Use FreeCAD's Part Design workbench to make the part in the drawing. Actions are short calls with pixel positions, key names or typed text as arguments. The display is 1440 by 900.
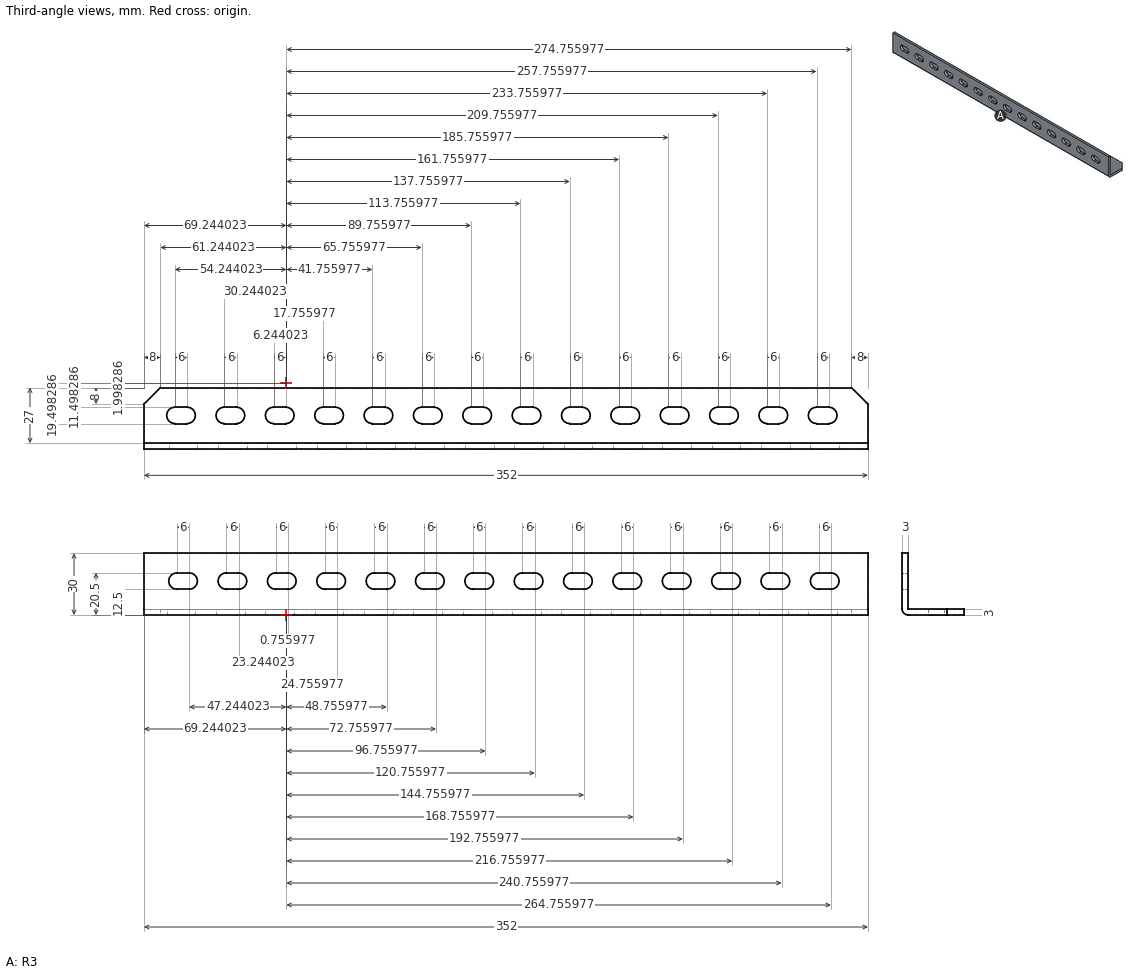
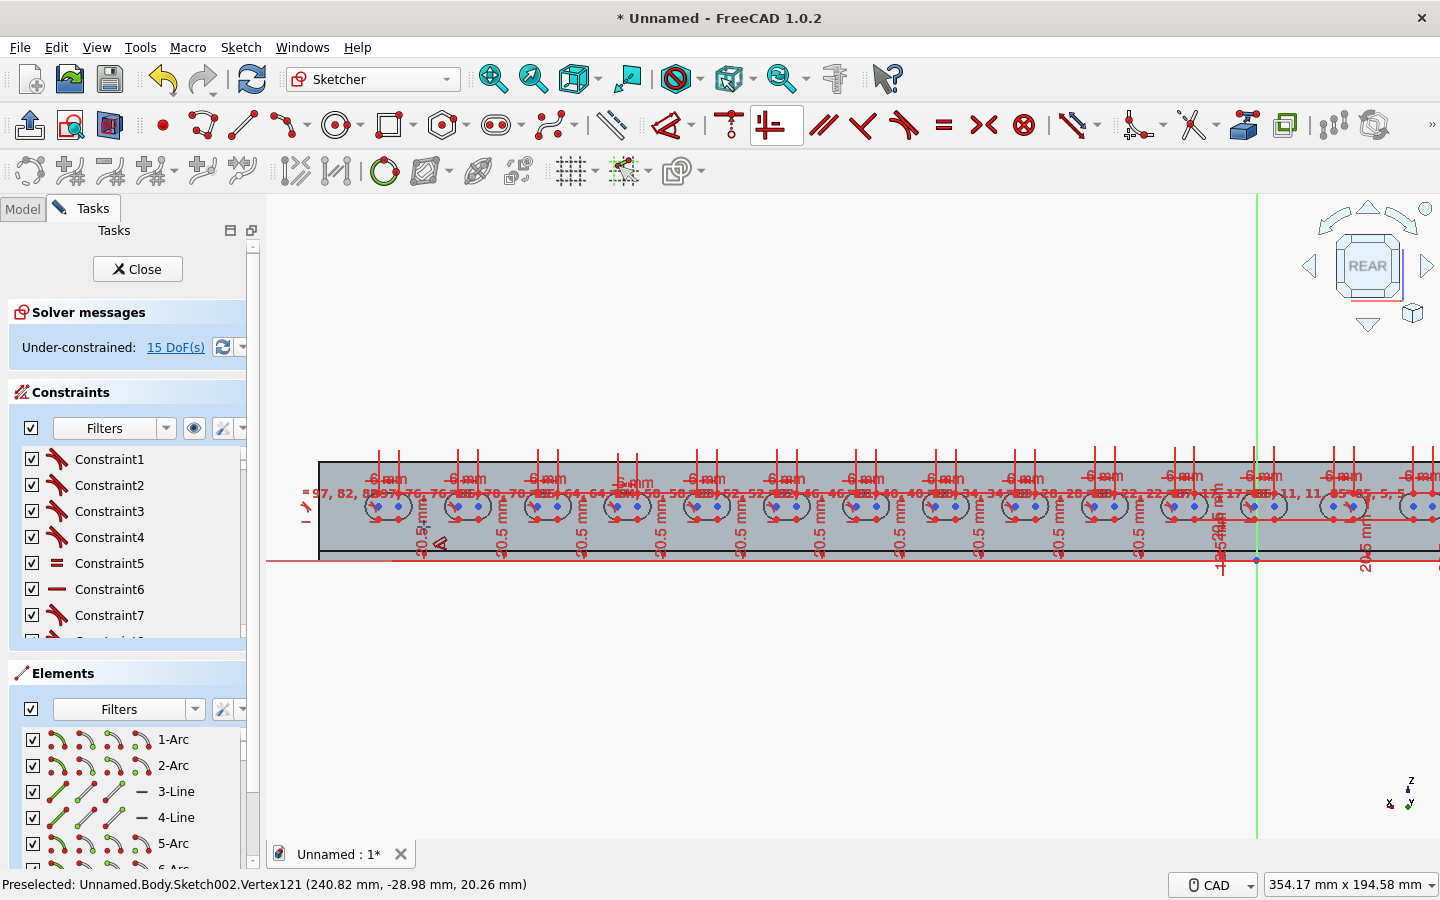
click(379, 493)
click(345, 527)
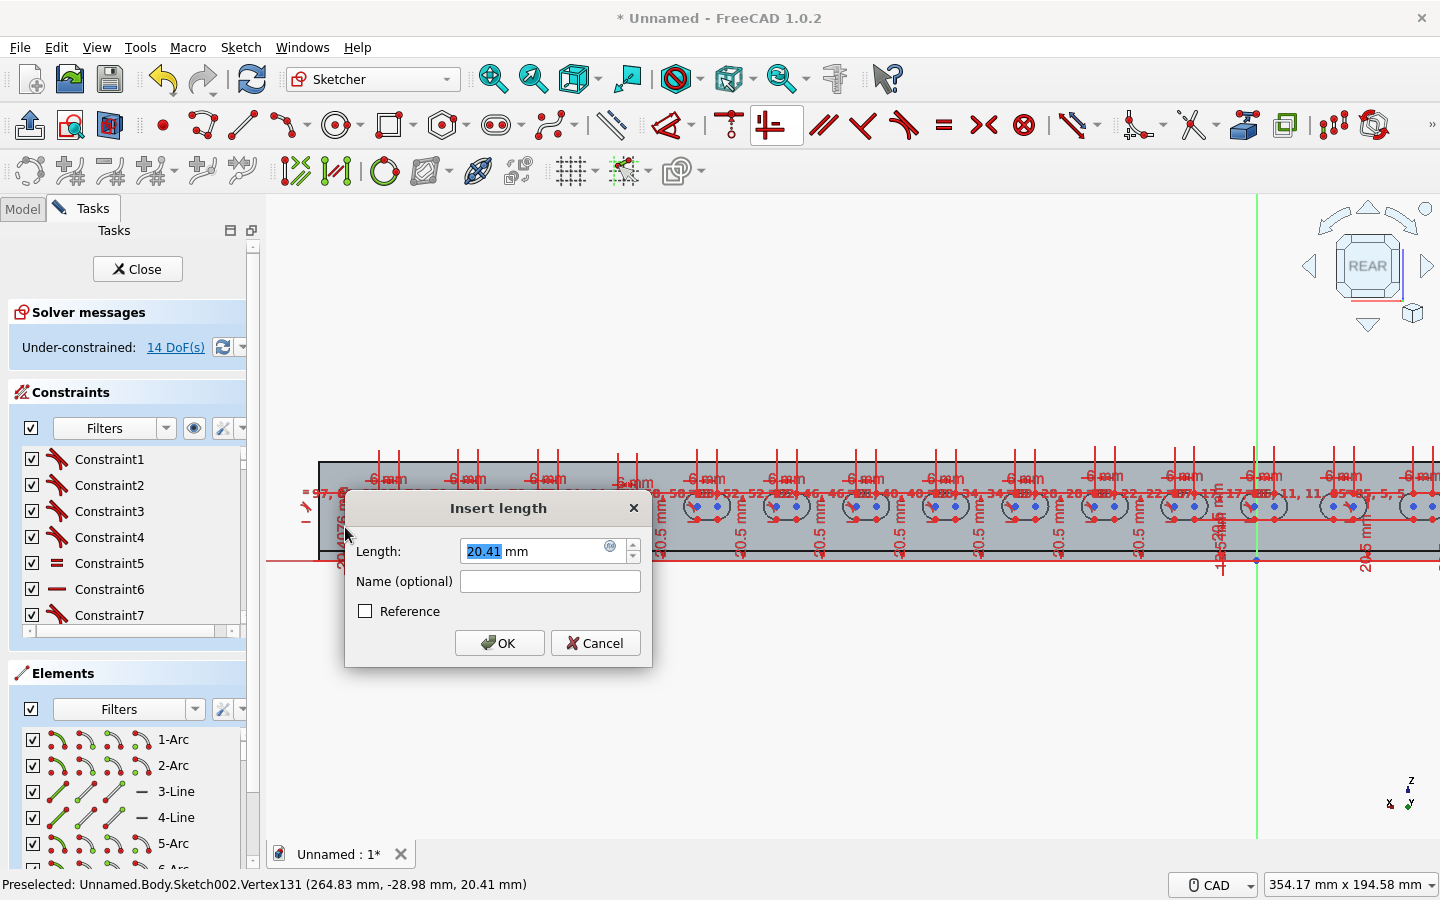
text(20.5)
key(Return)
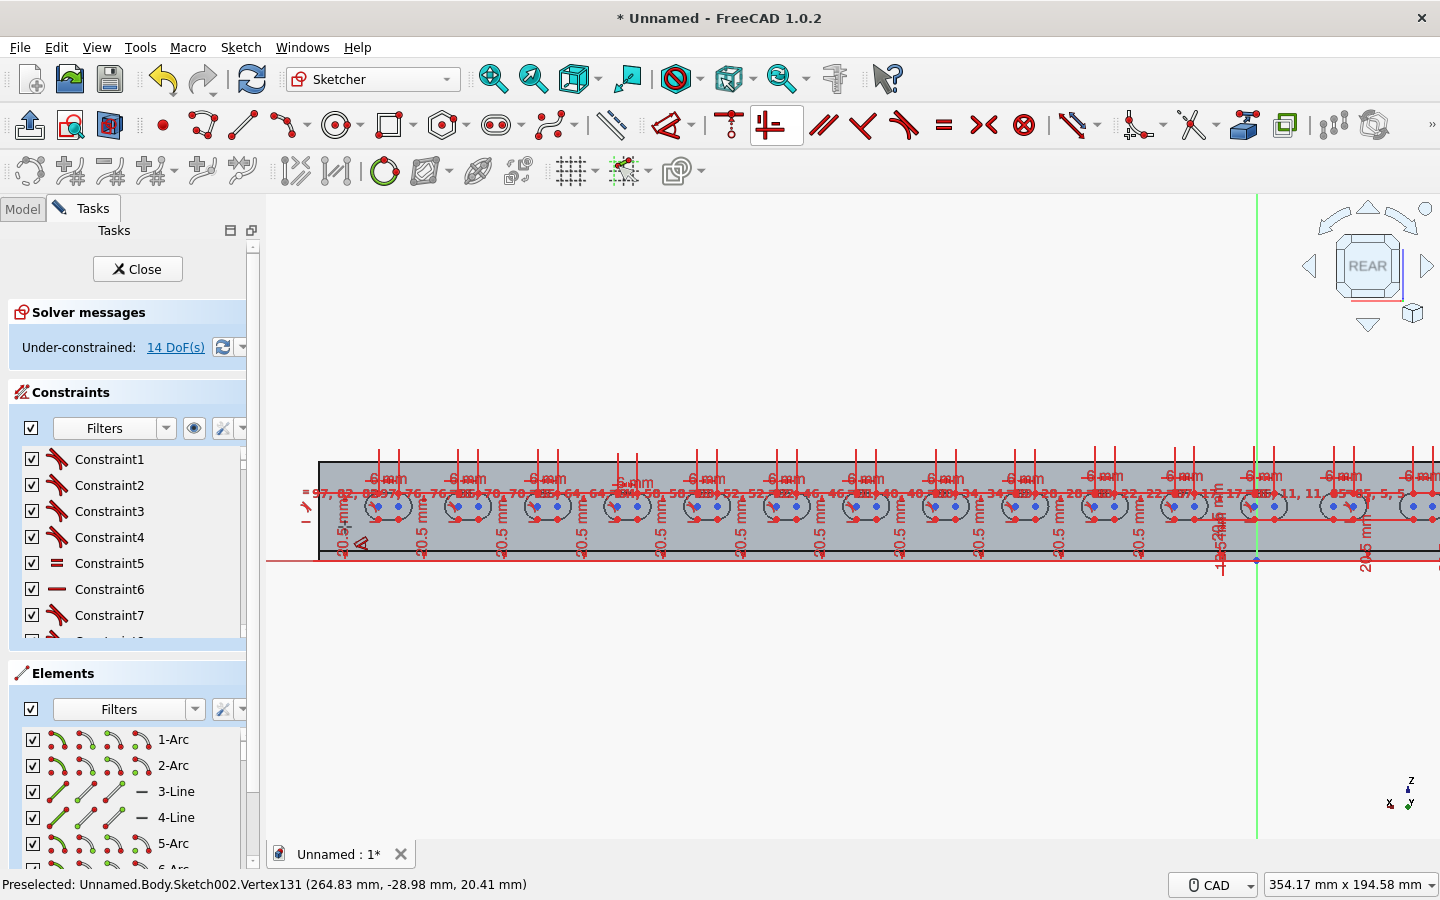
scroll(1254, 493, up, 14)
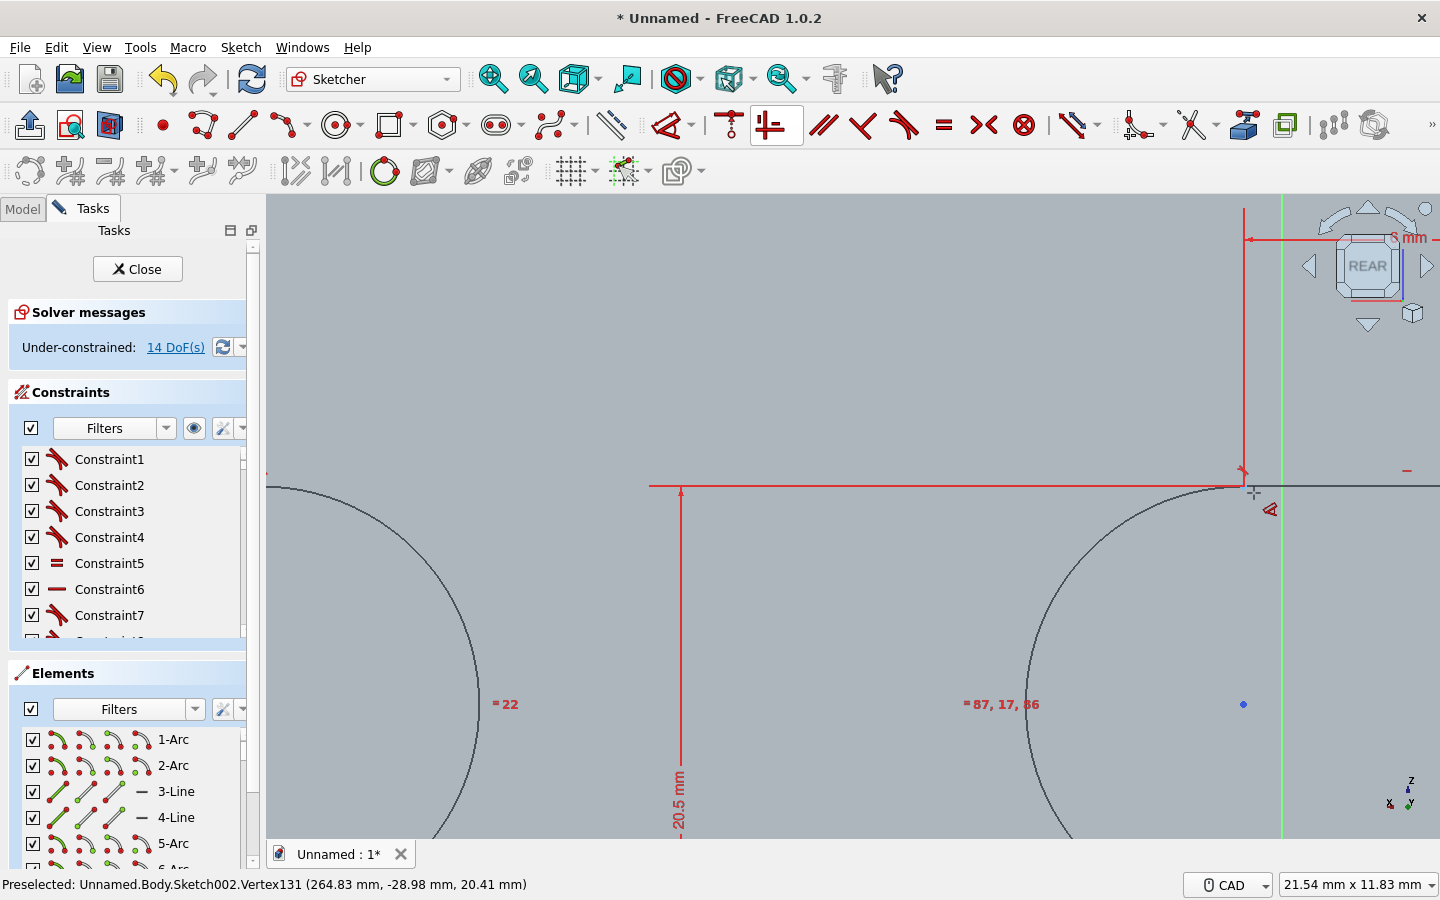
click(1244, 486)
click(1259, 452)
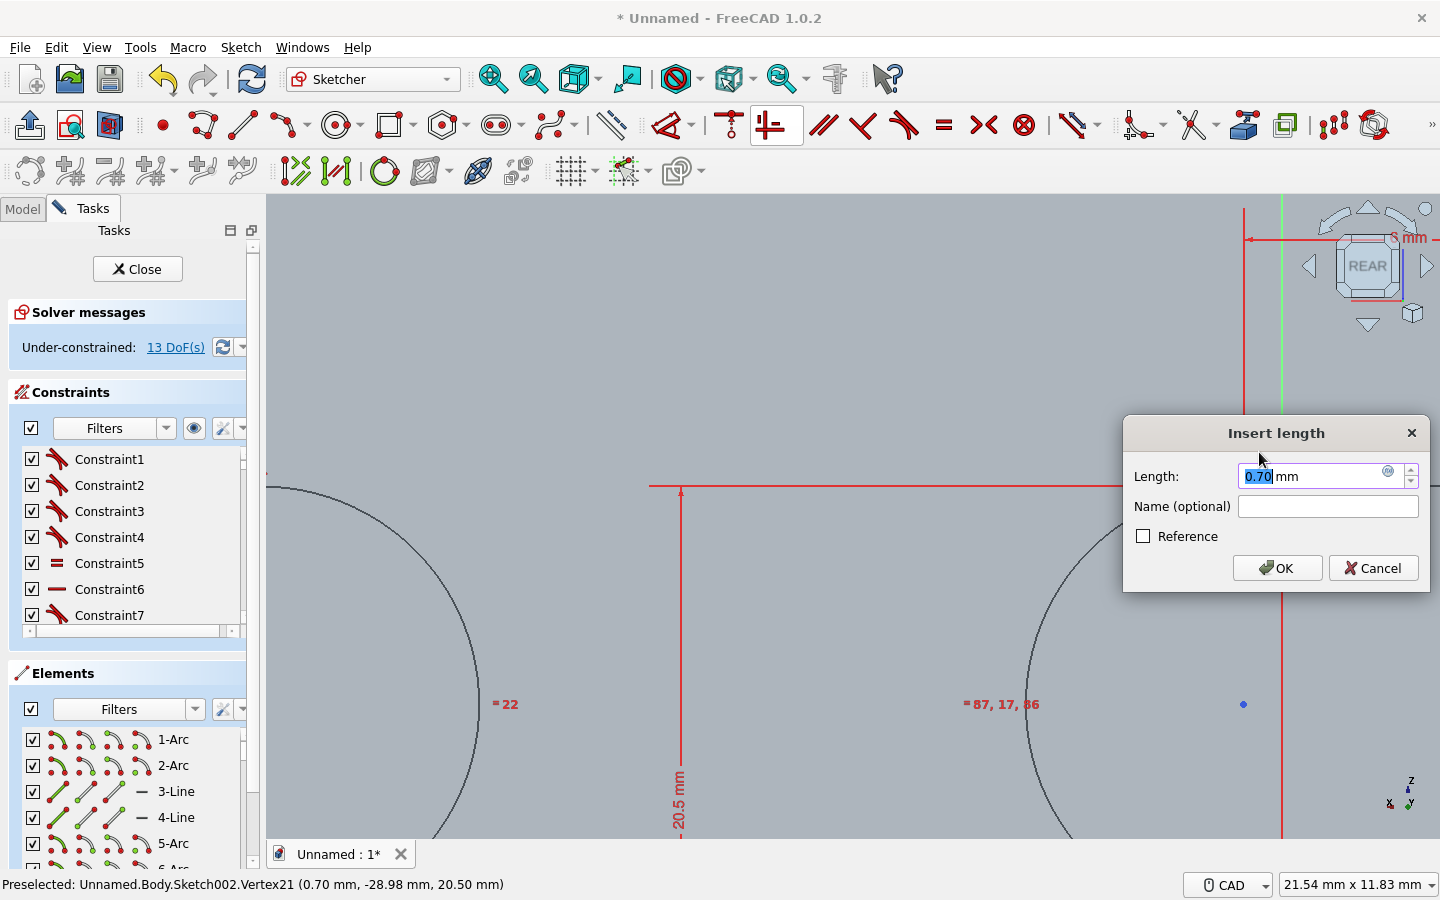
text(0.755977)
key(Return)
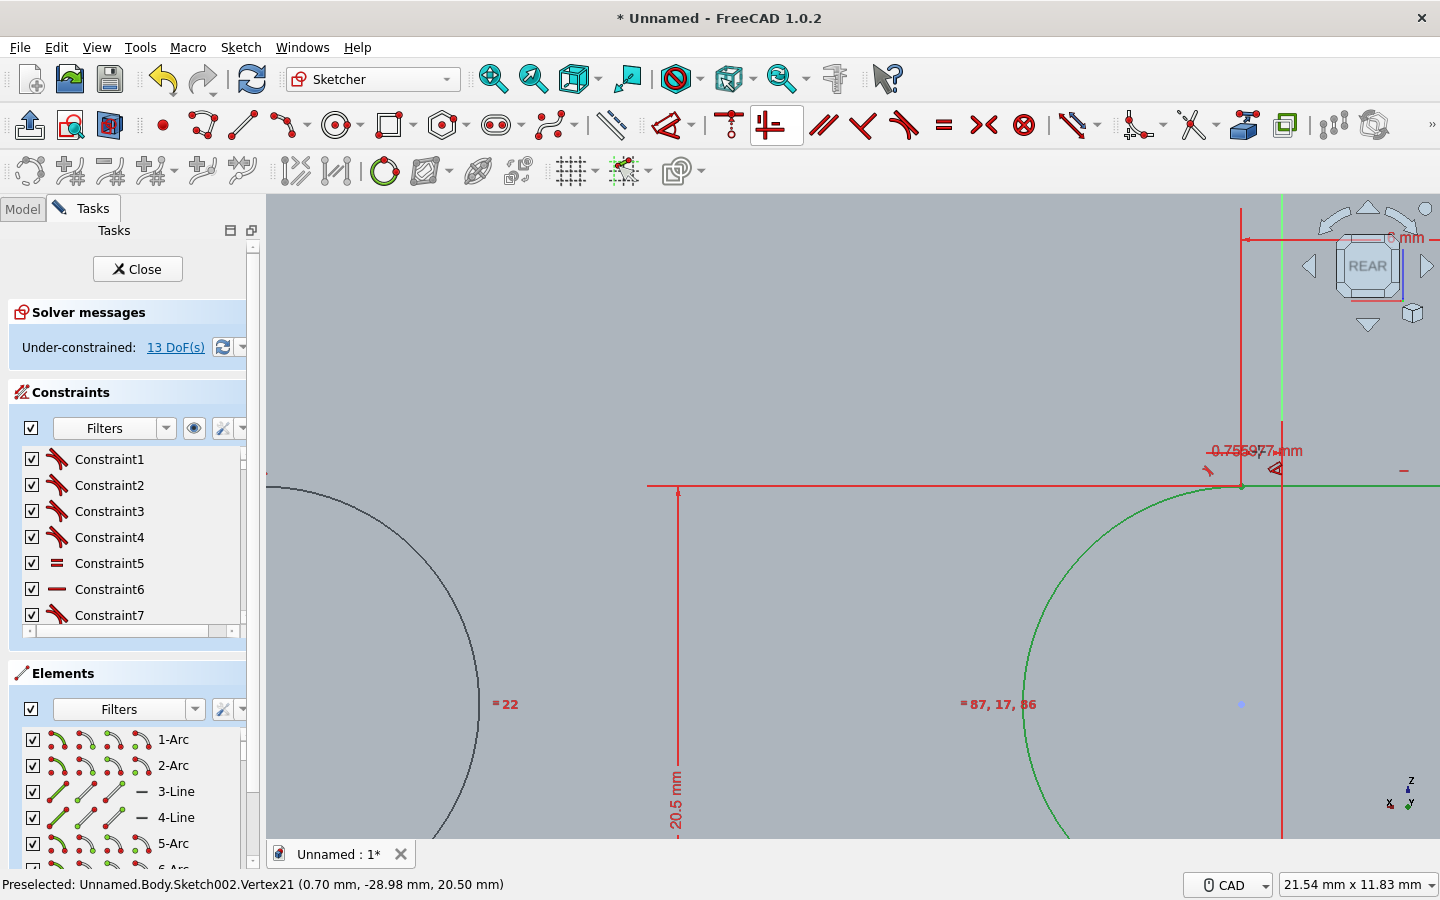
scroll(1060, 489, down, 15)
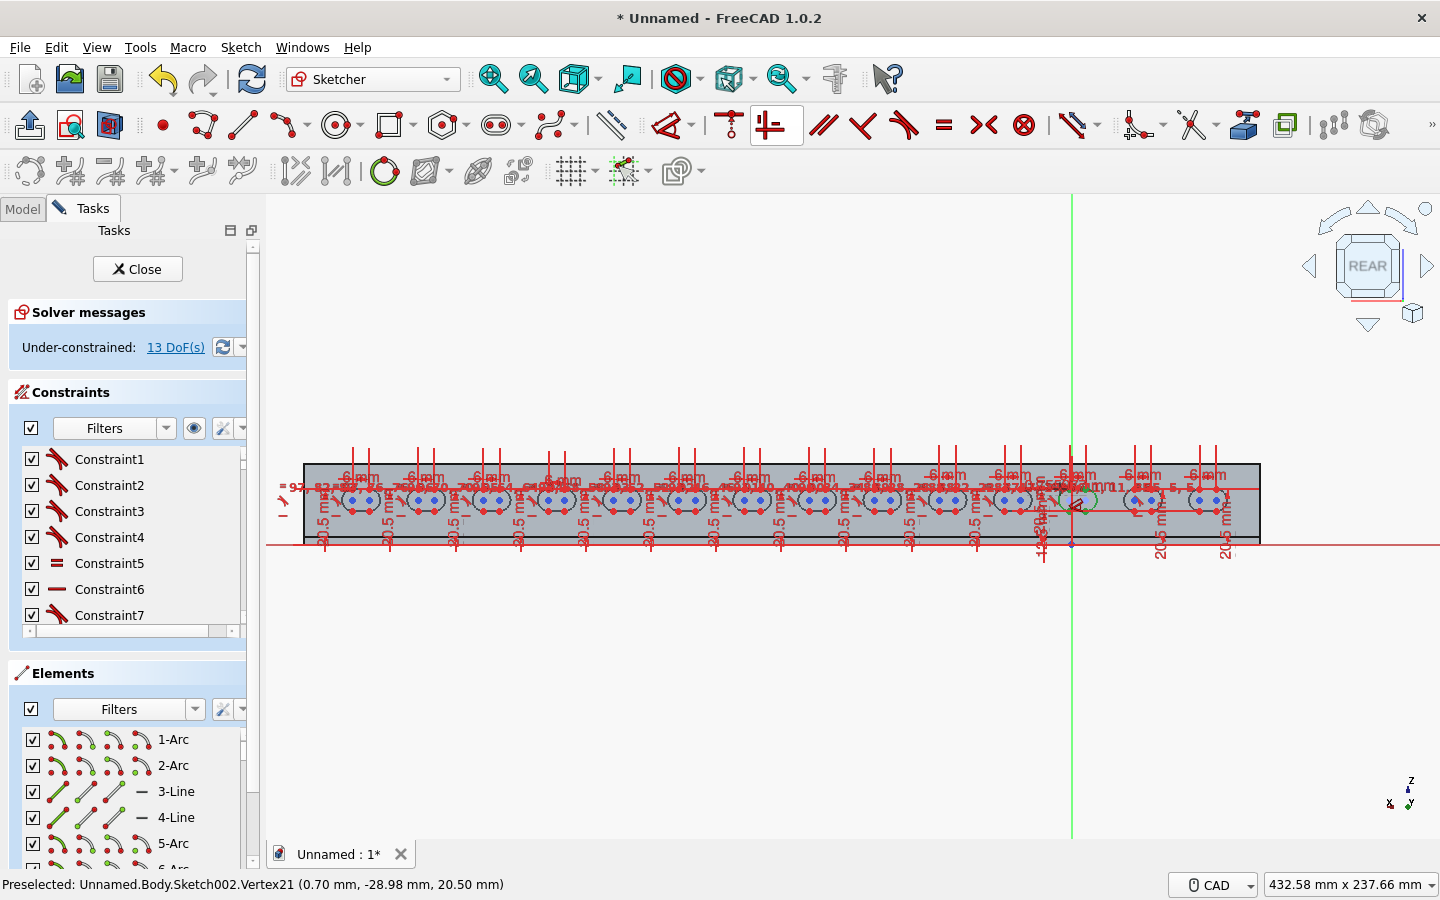
click(1200, 489)
click(1136, 579)